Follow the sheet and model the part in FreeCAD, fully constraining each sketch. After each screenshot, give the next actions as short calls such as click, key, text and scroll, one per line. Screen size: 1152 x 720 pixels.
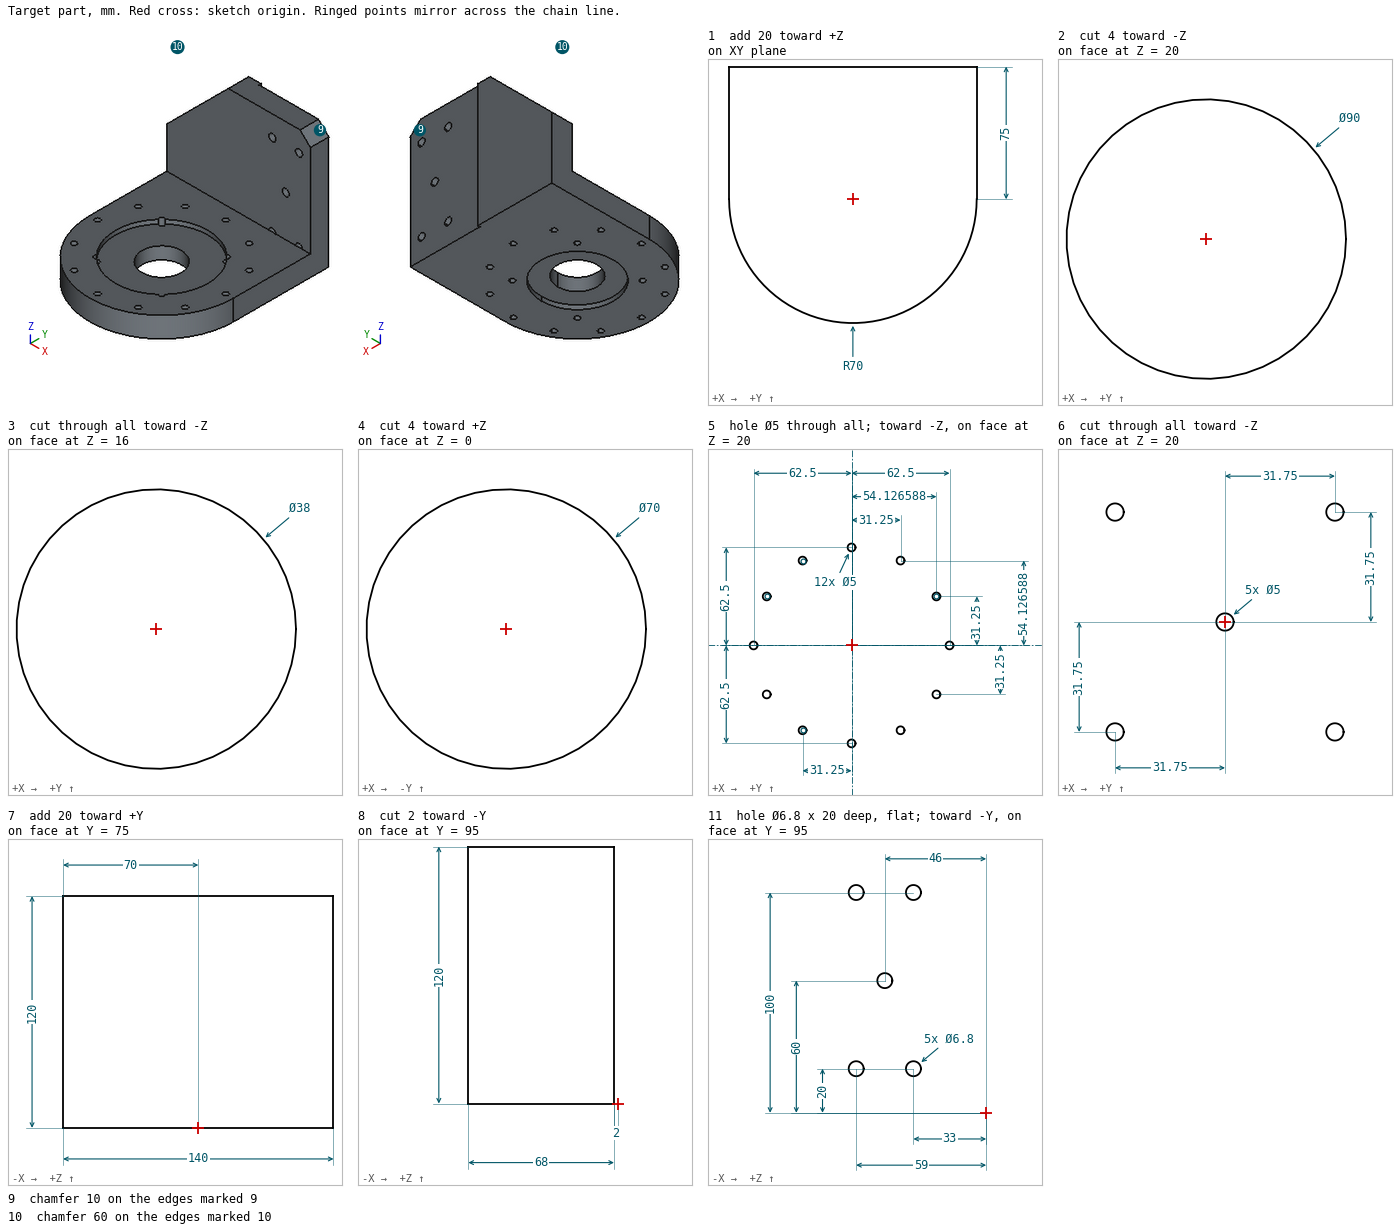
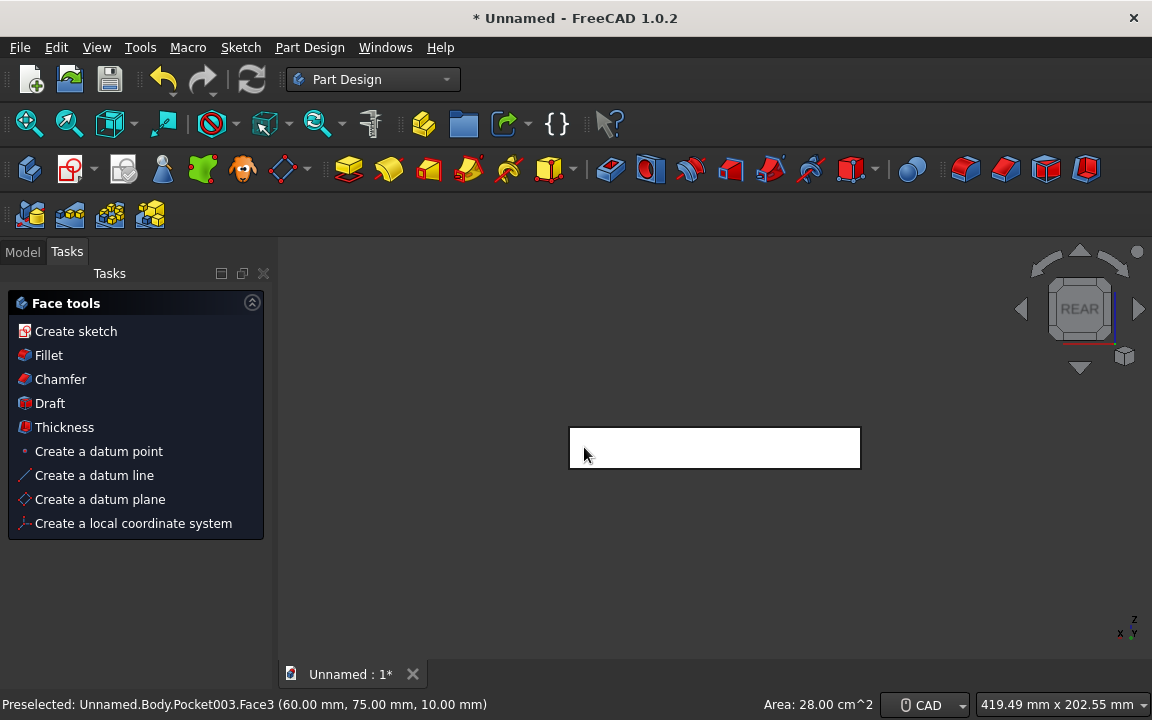
click(70, 170)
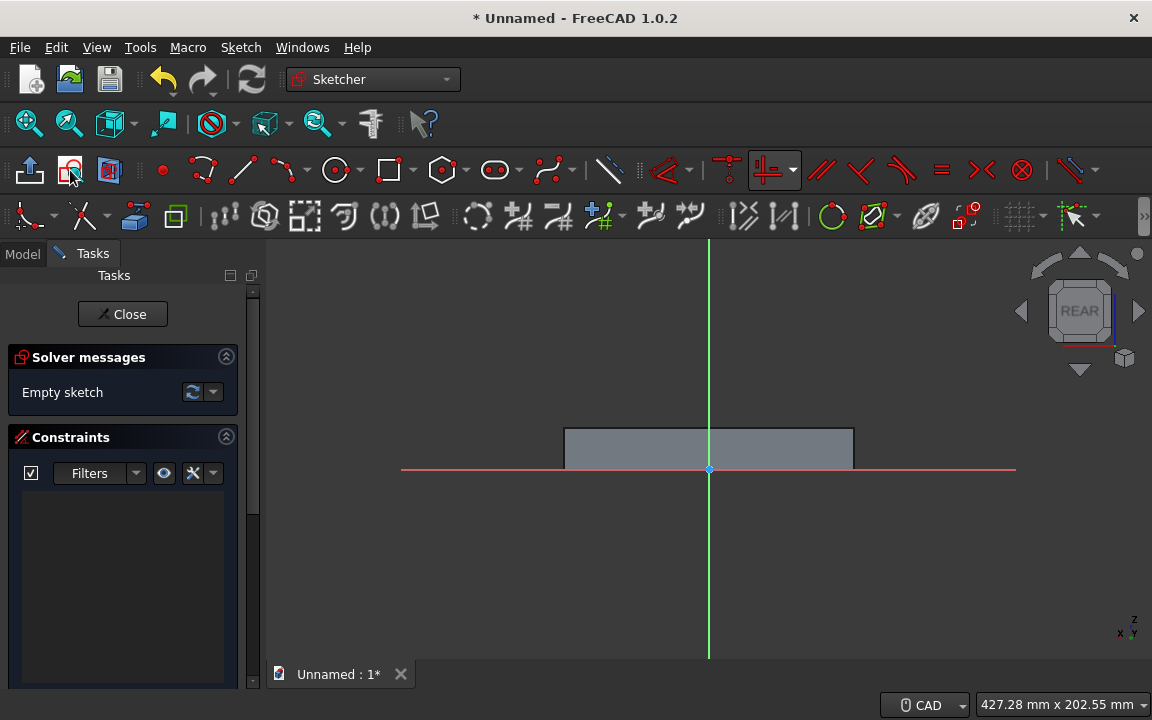
scroll(331, 631, down, 1)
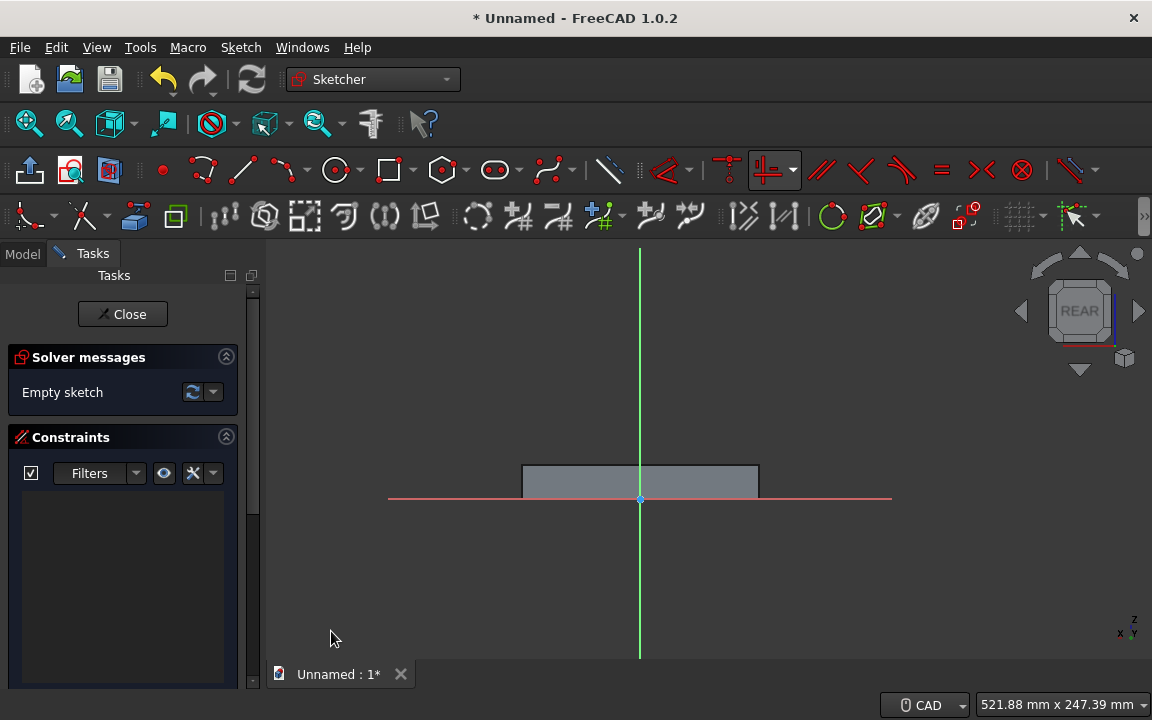
key(g)
key(r)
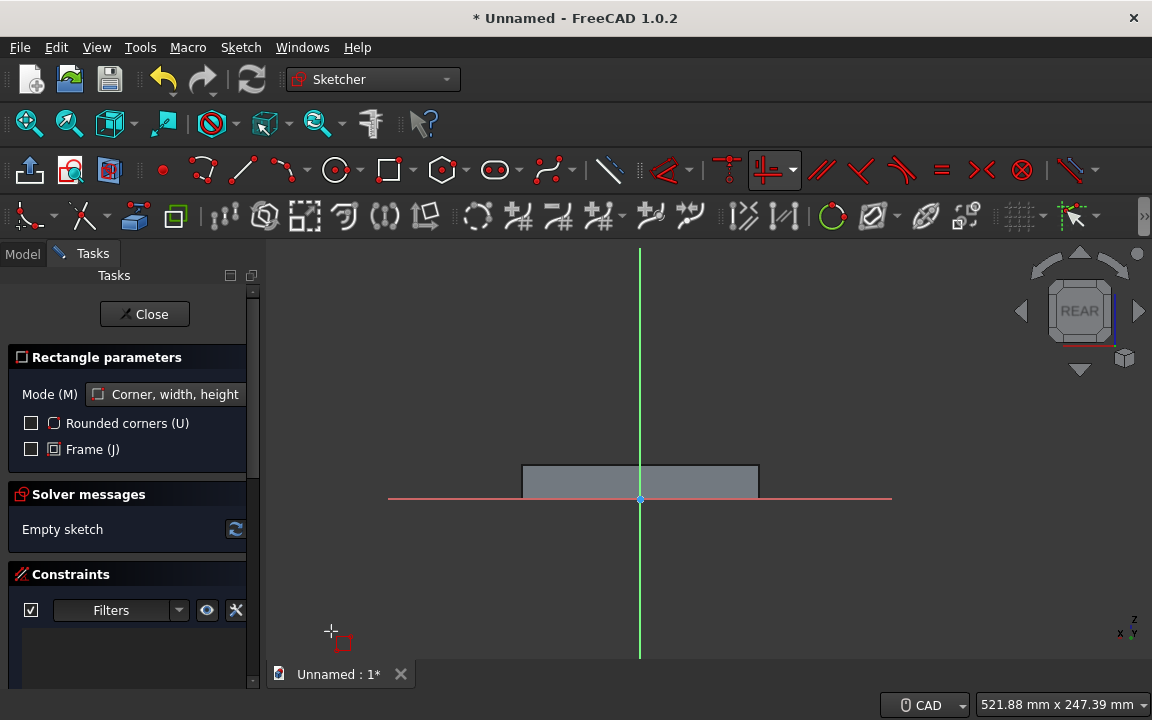
click(522, 295)
click(759, 499)
key(Escape)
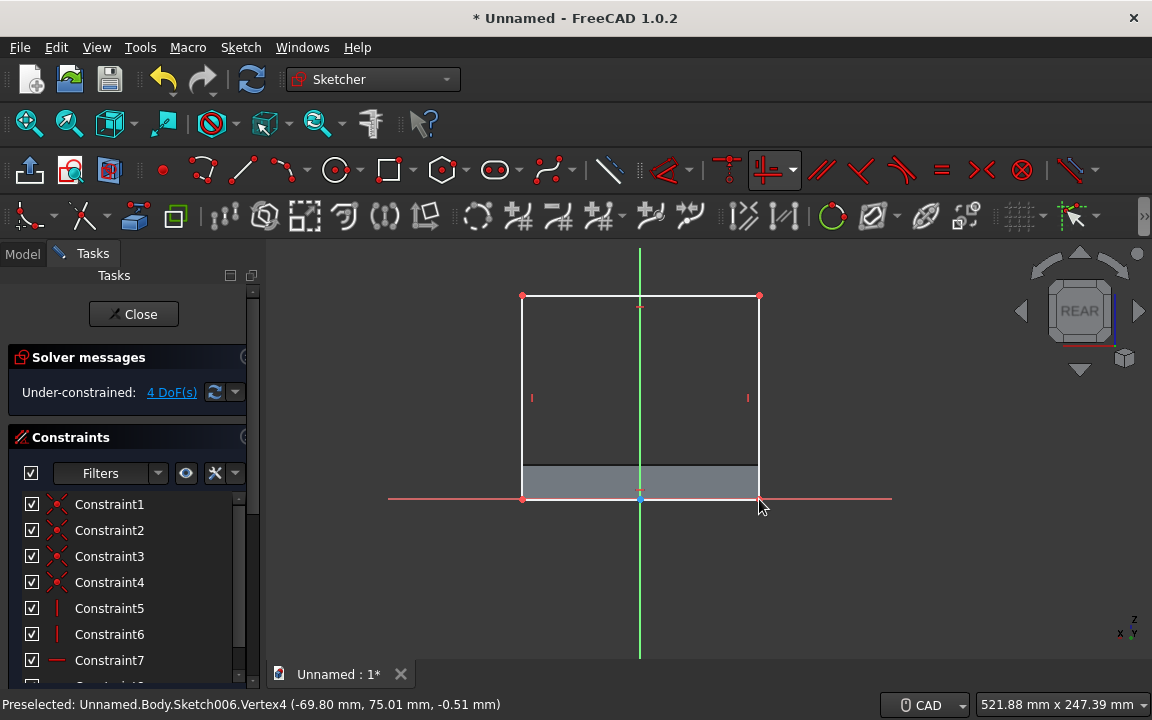
click(522, 500)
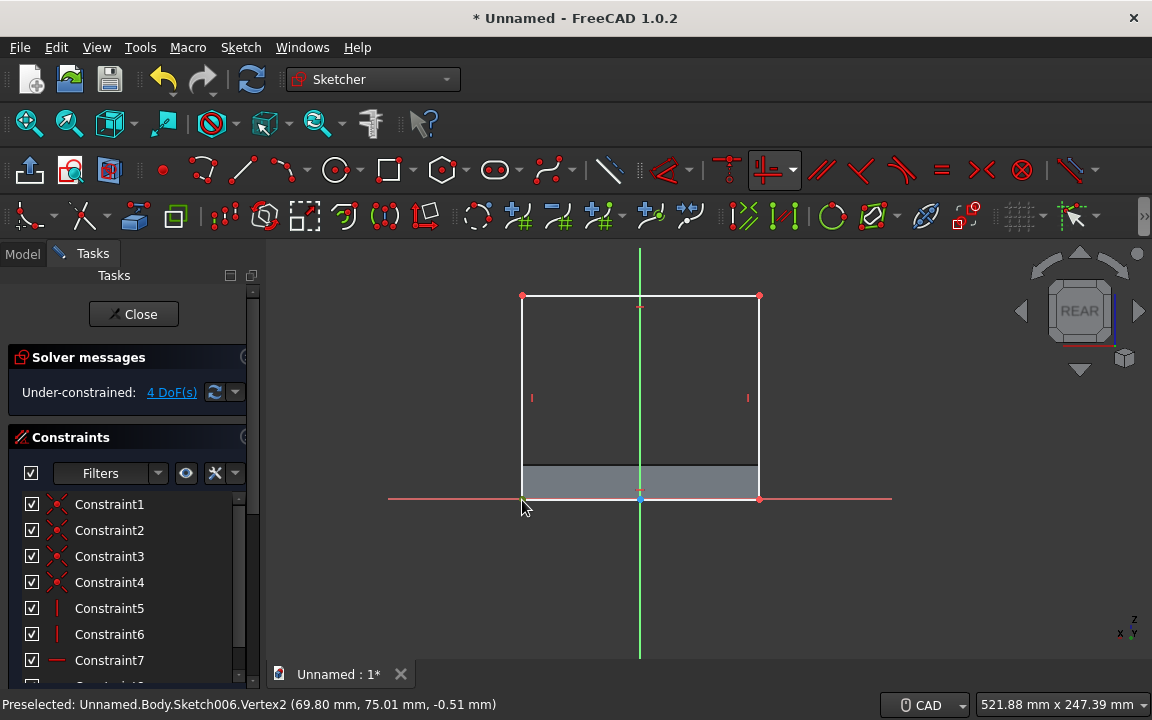
click(393, 499)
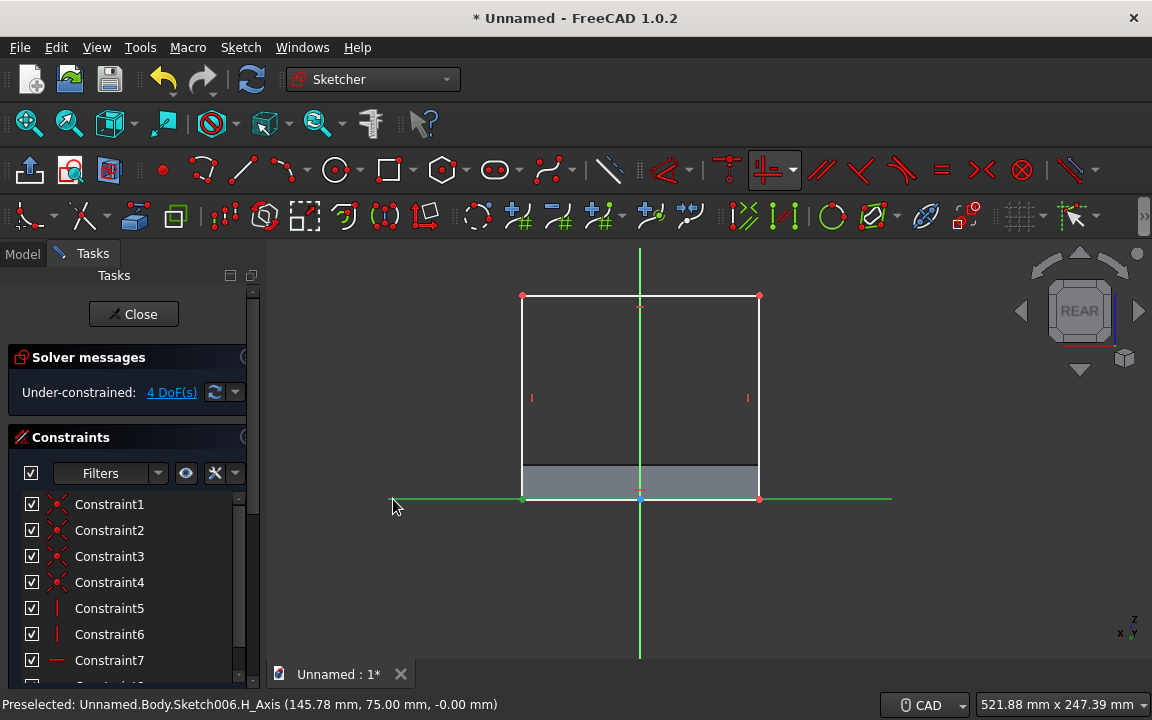
key(c)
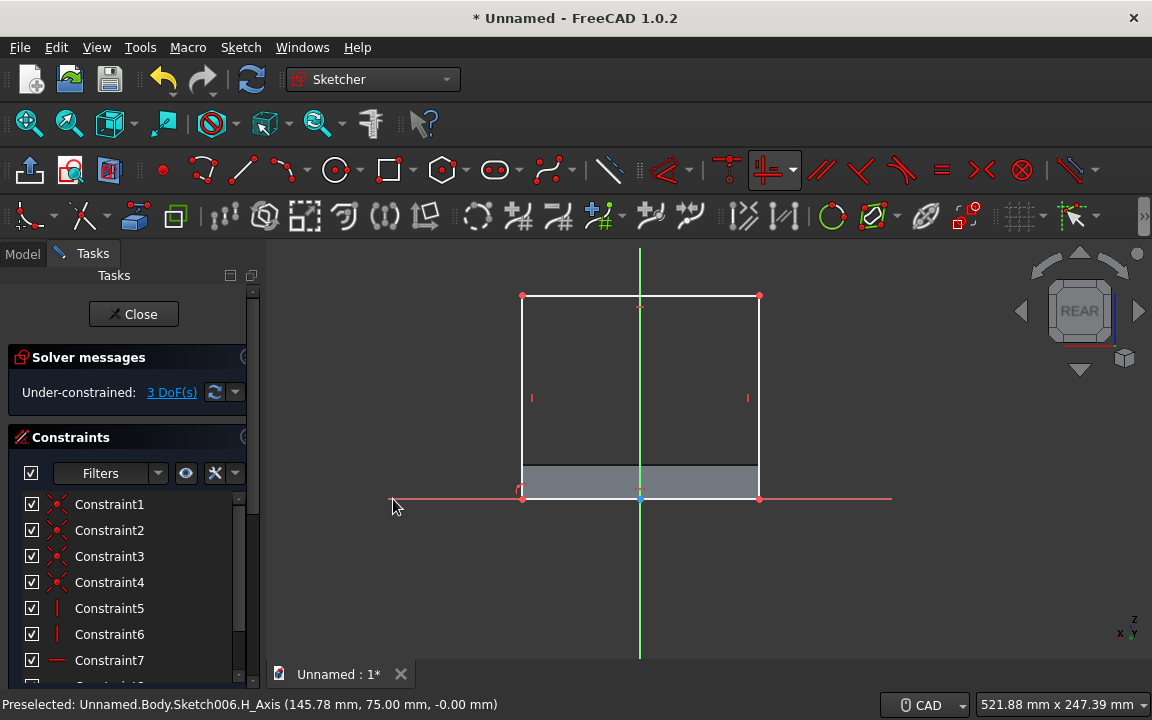
key(d)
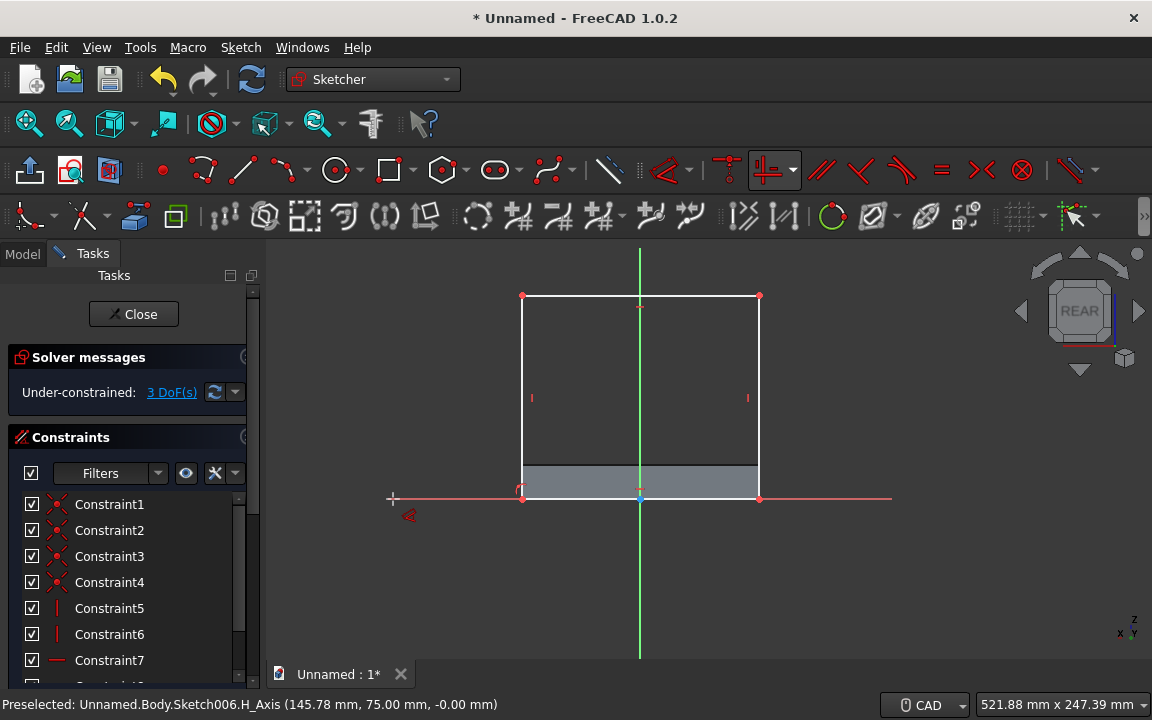
click(522, 357)
click(488, 398)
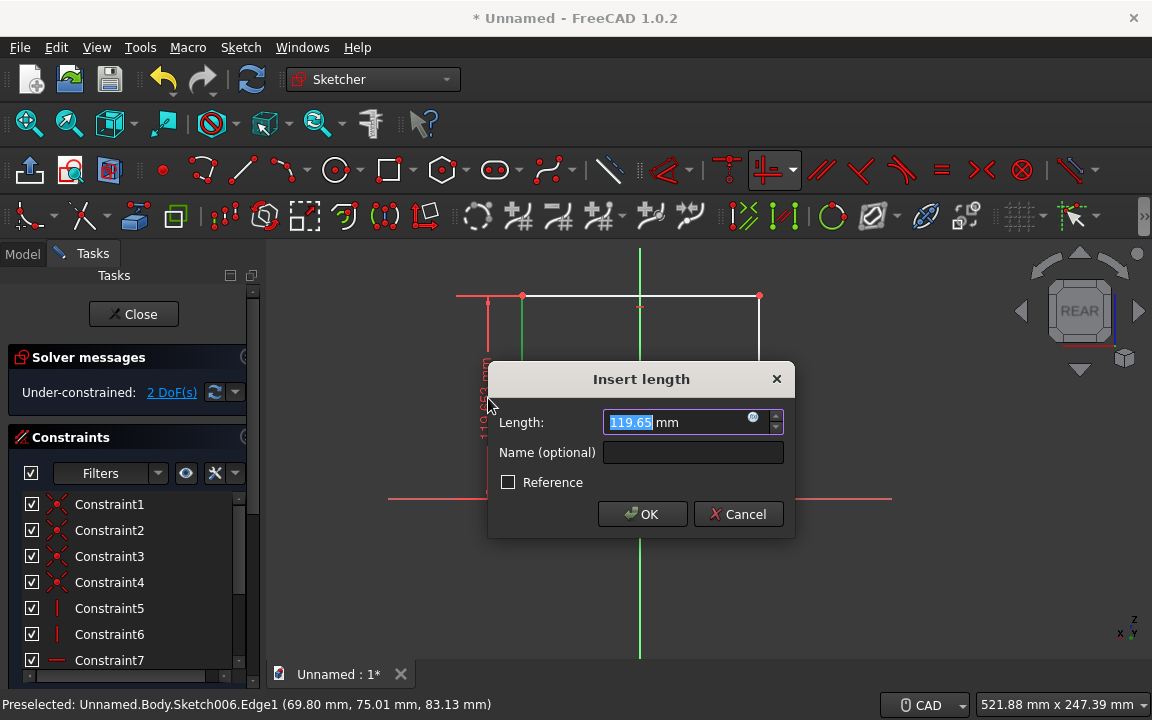
text(120)
key(Return)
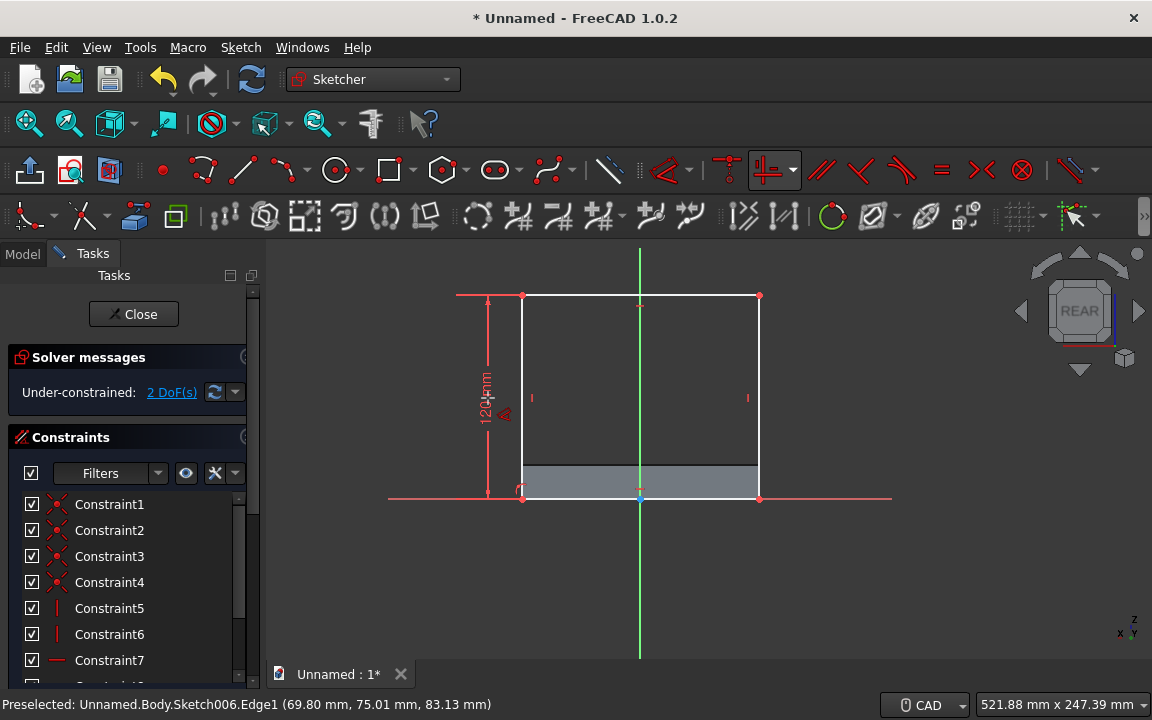
click(593, 499)
click(586, 533)